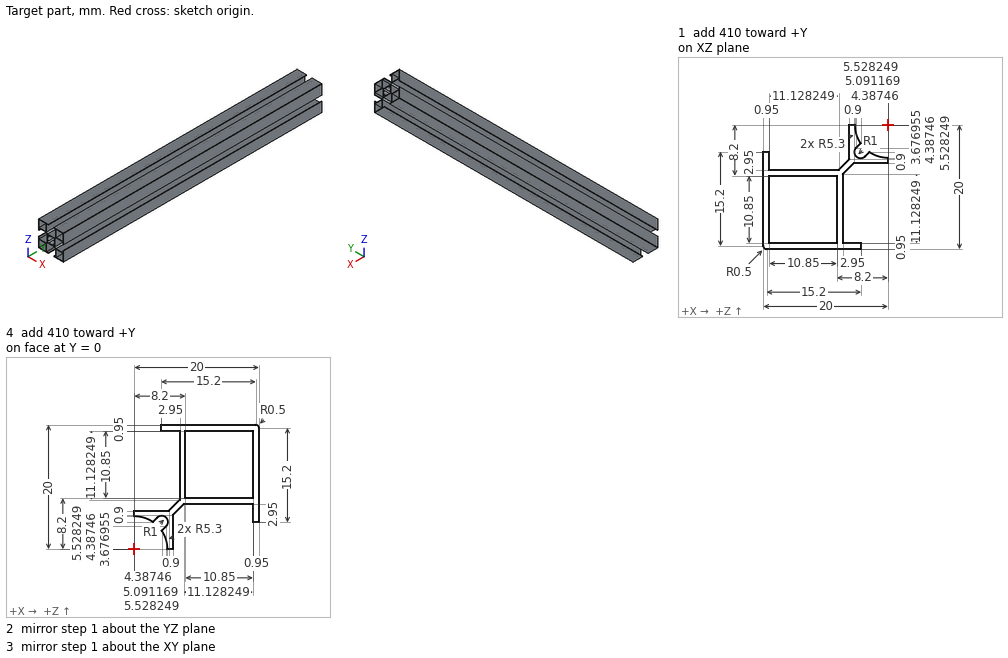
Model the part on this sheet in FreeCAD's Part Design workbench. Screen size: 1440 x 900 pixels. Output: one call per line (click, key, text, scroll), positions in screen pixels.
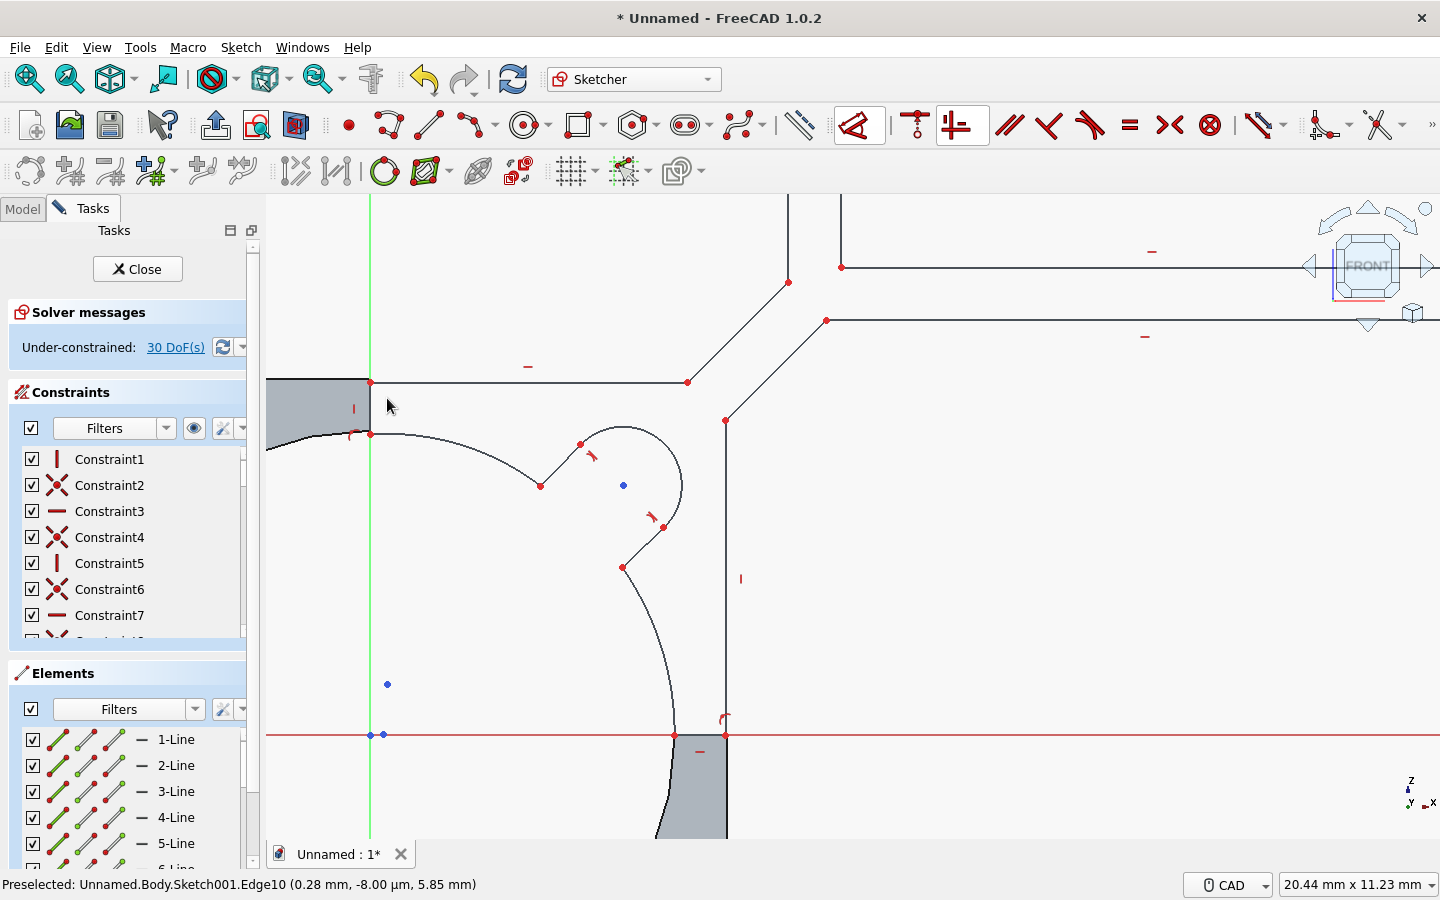
click(670, 682)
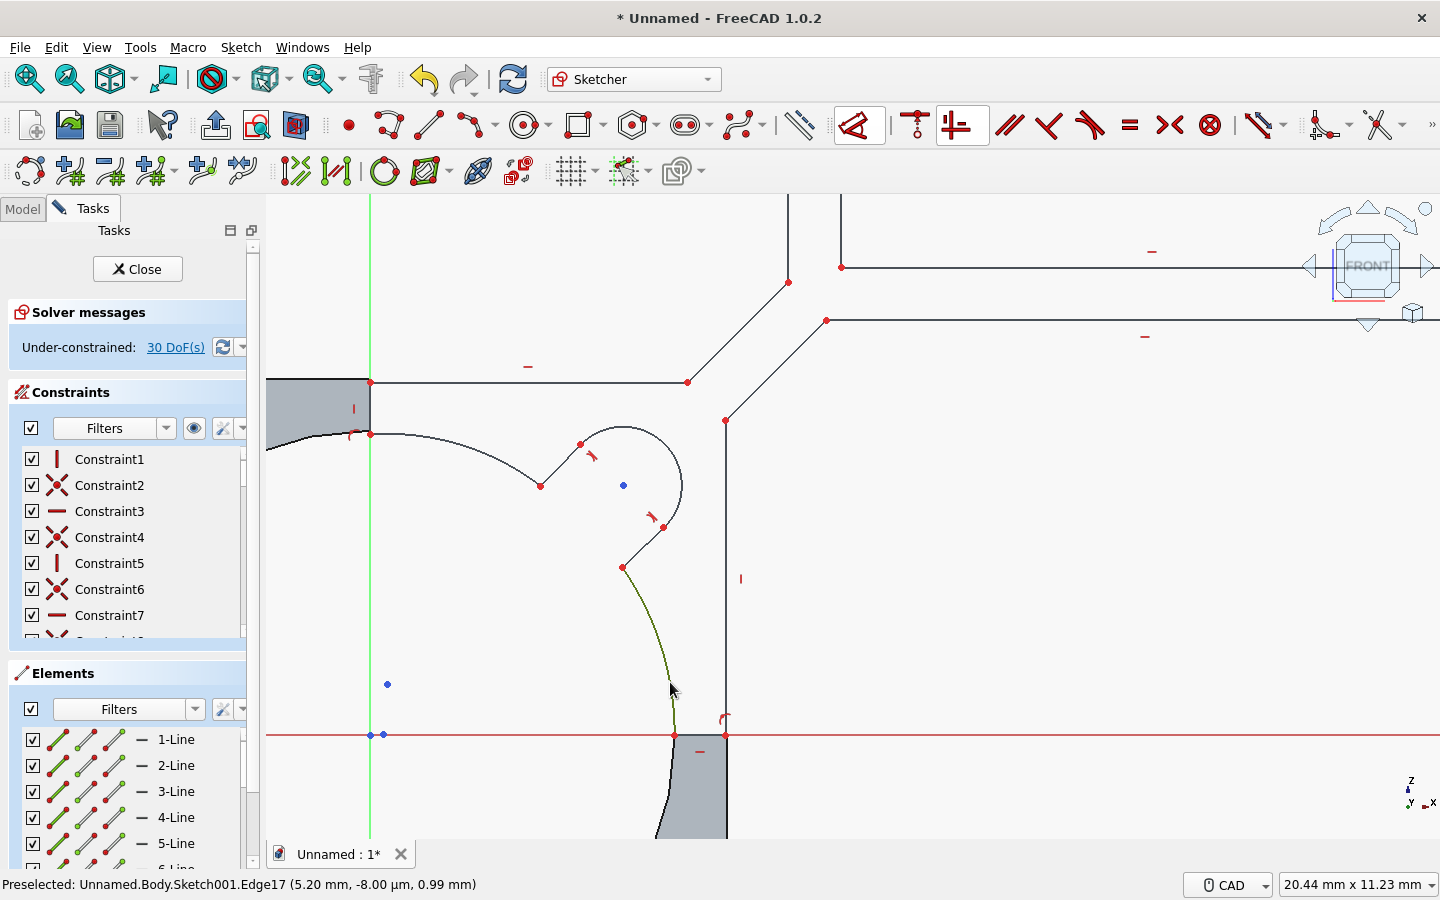
click(494, 458)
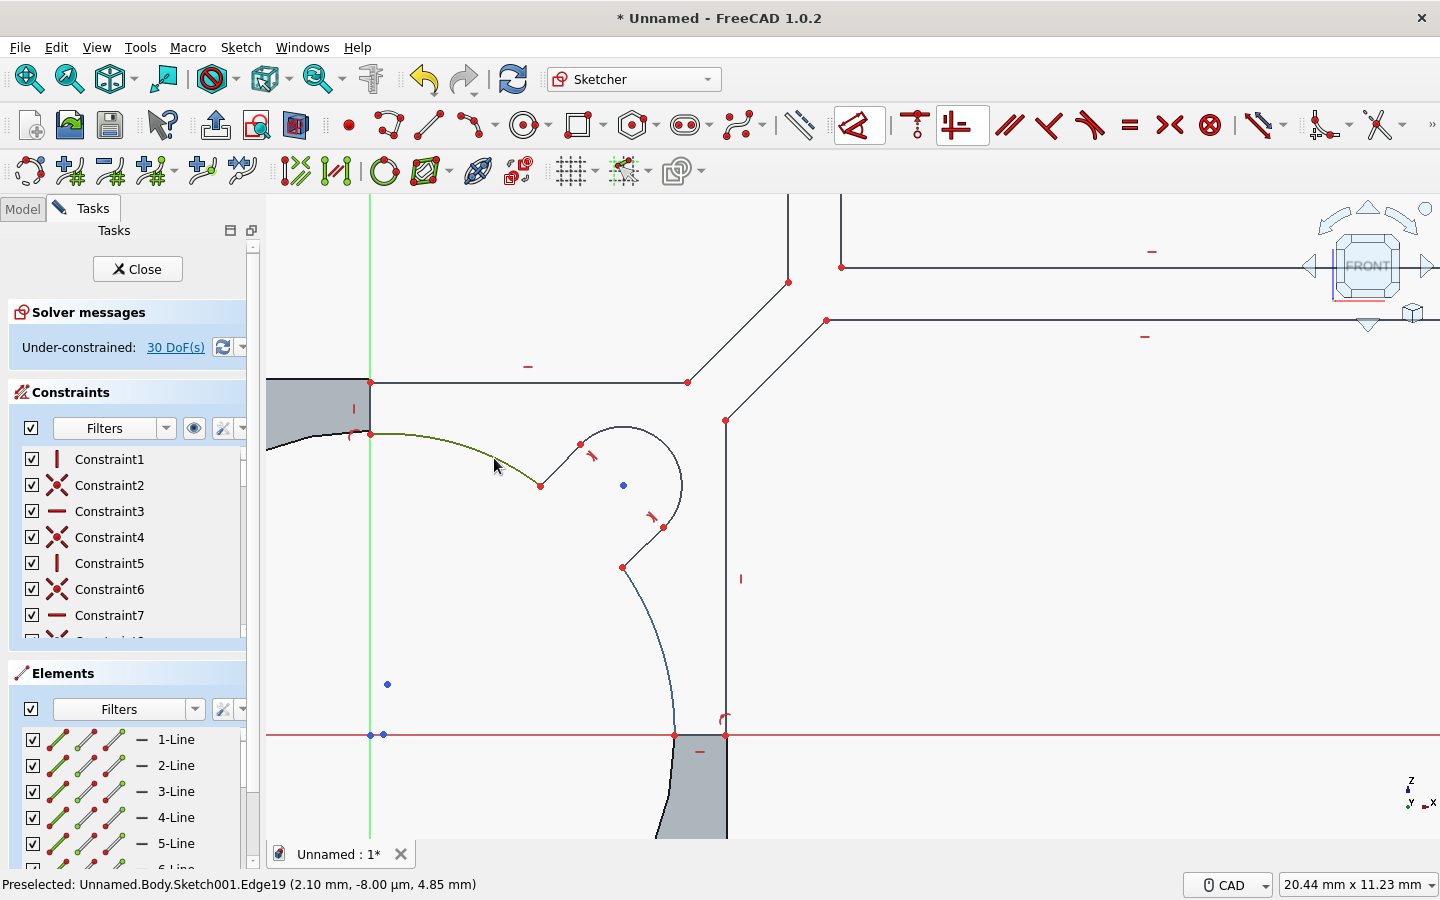
click(916, 126)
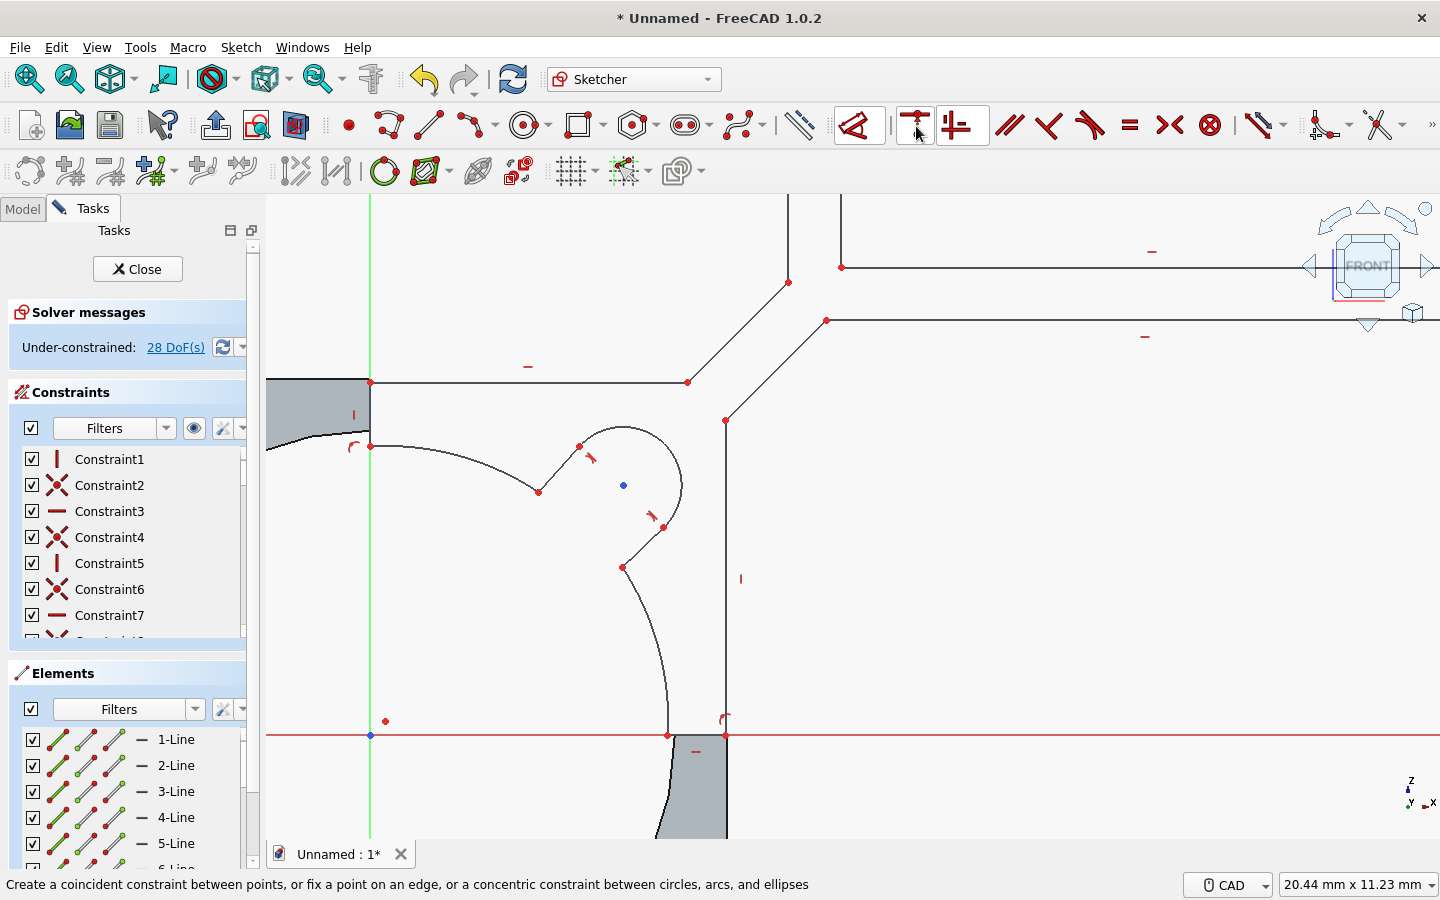
scroll(378, 728, up, 2)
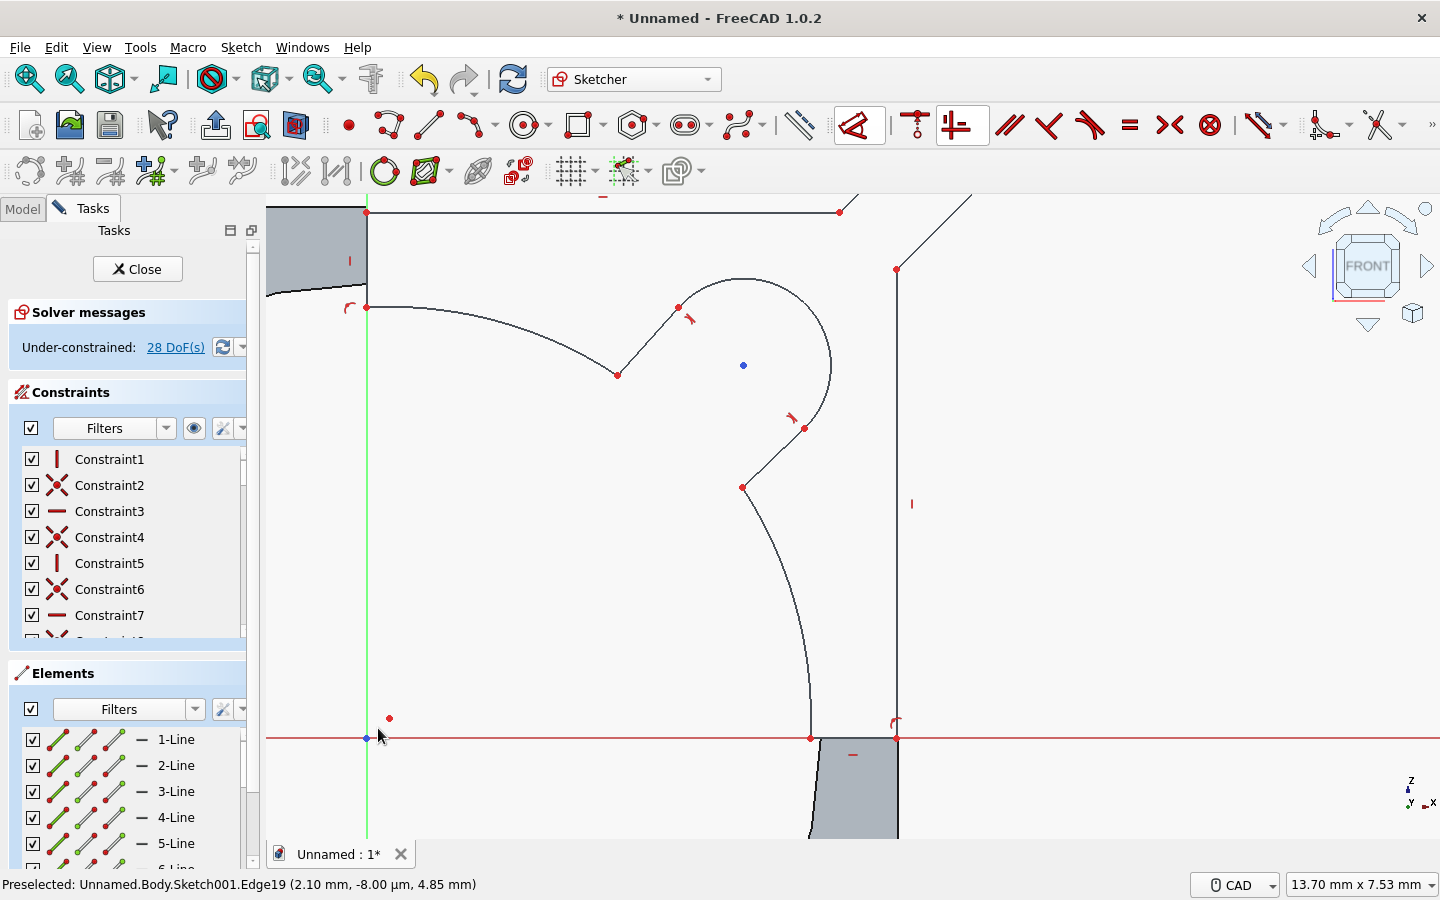
drag(357, 708, 400, 748)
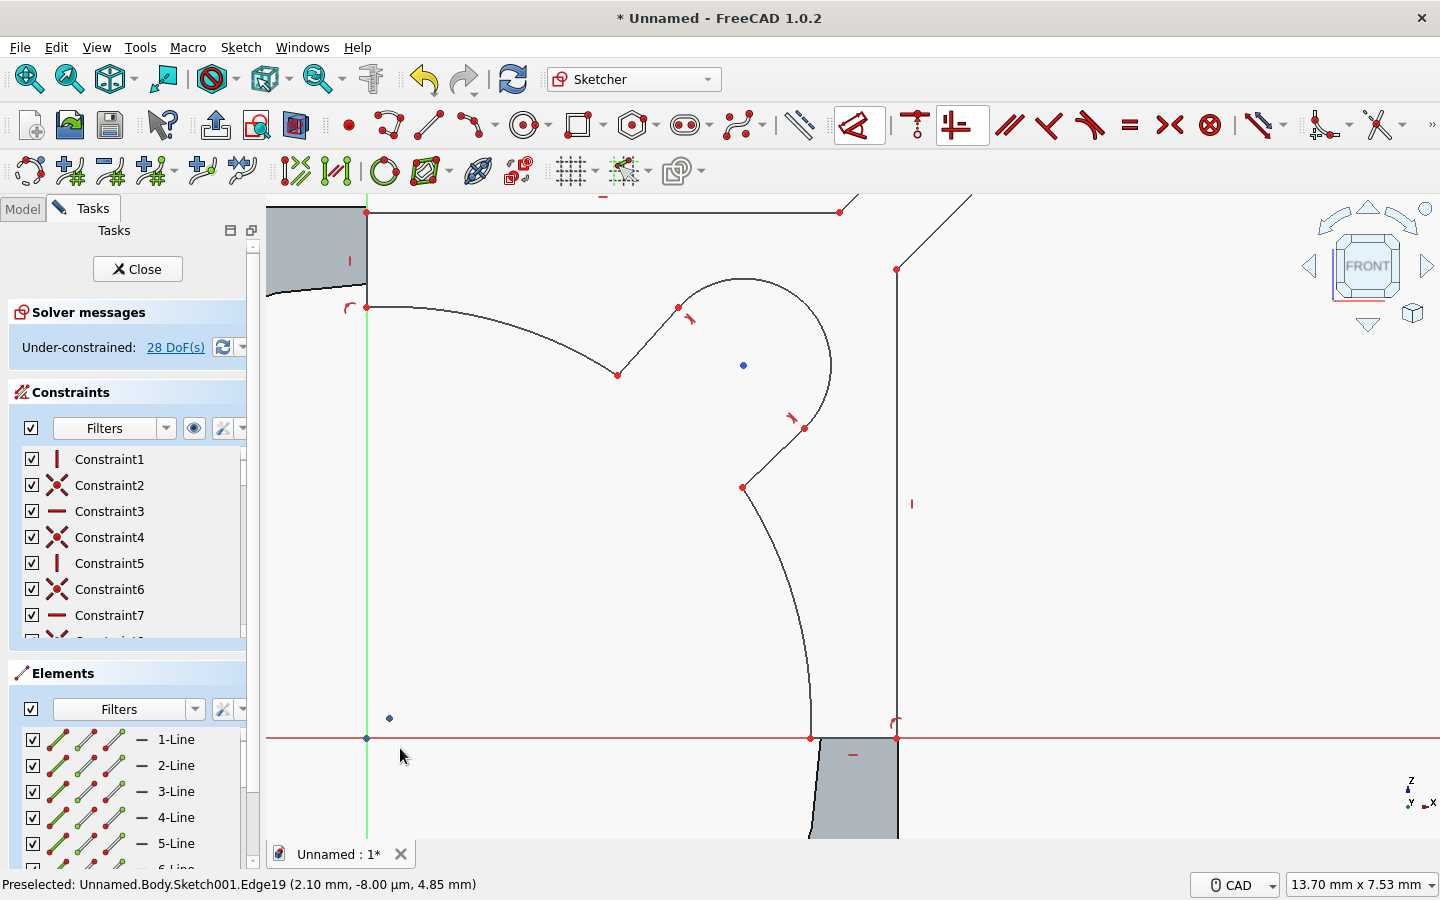
click(916, 126)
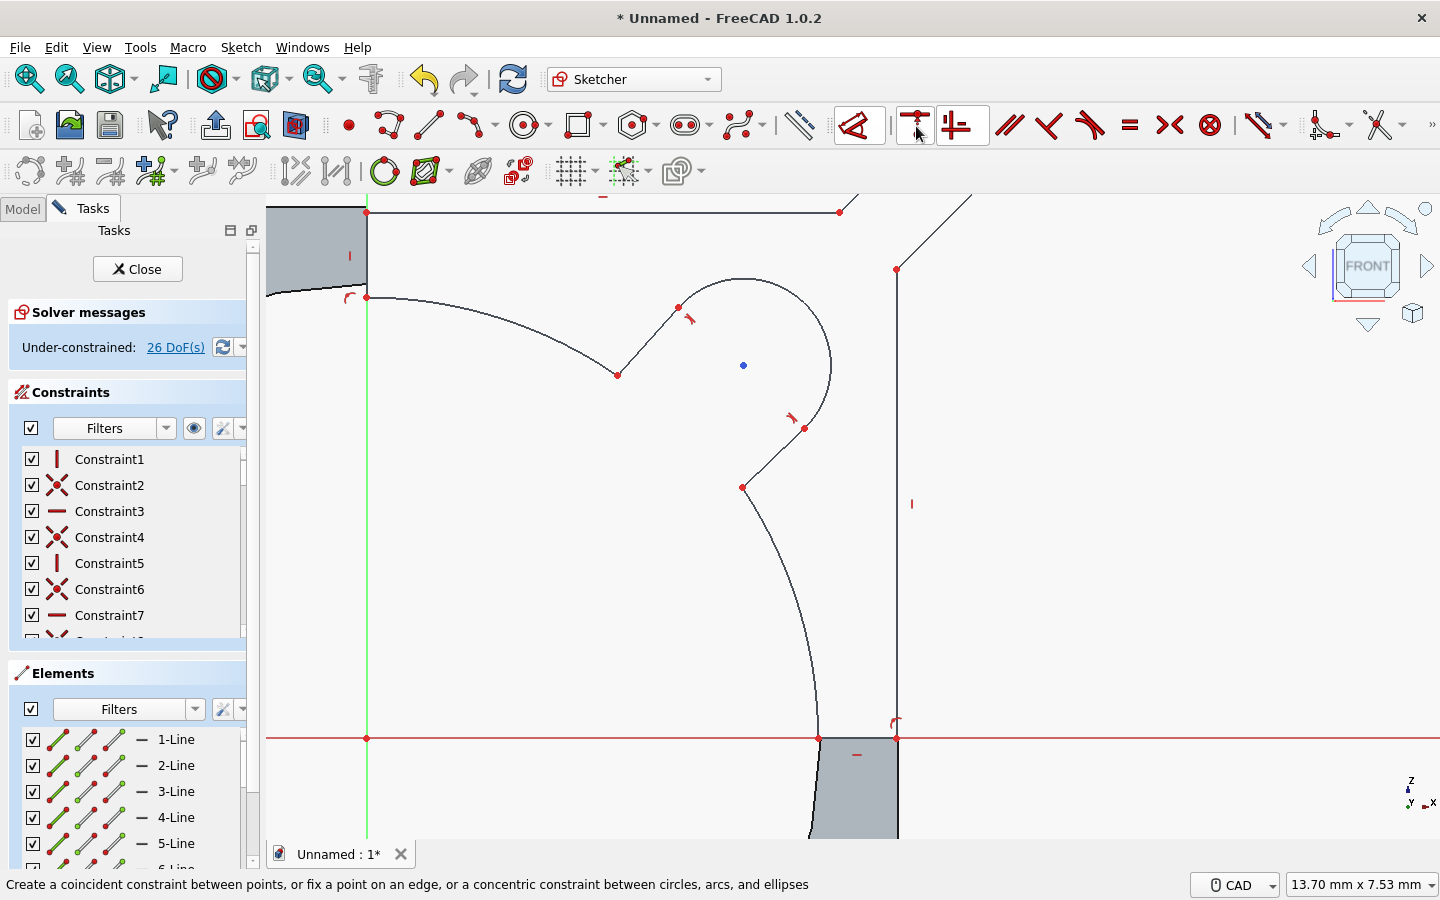
scroll(641, 724, down, 7)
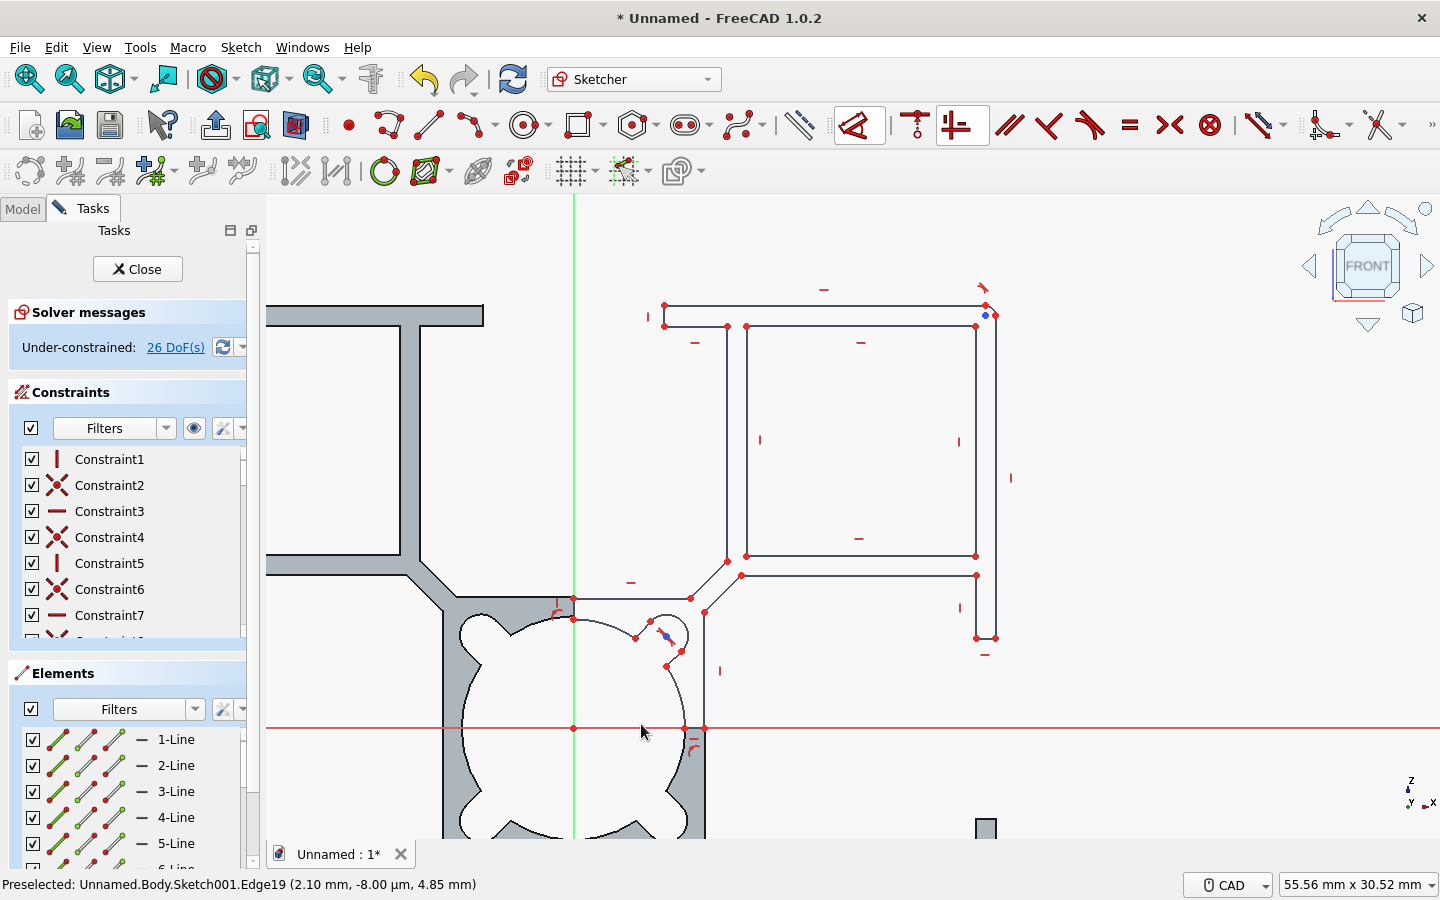
click(683, 709)